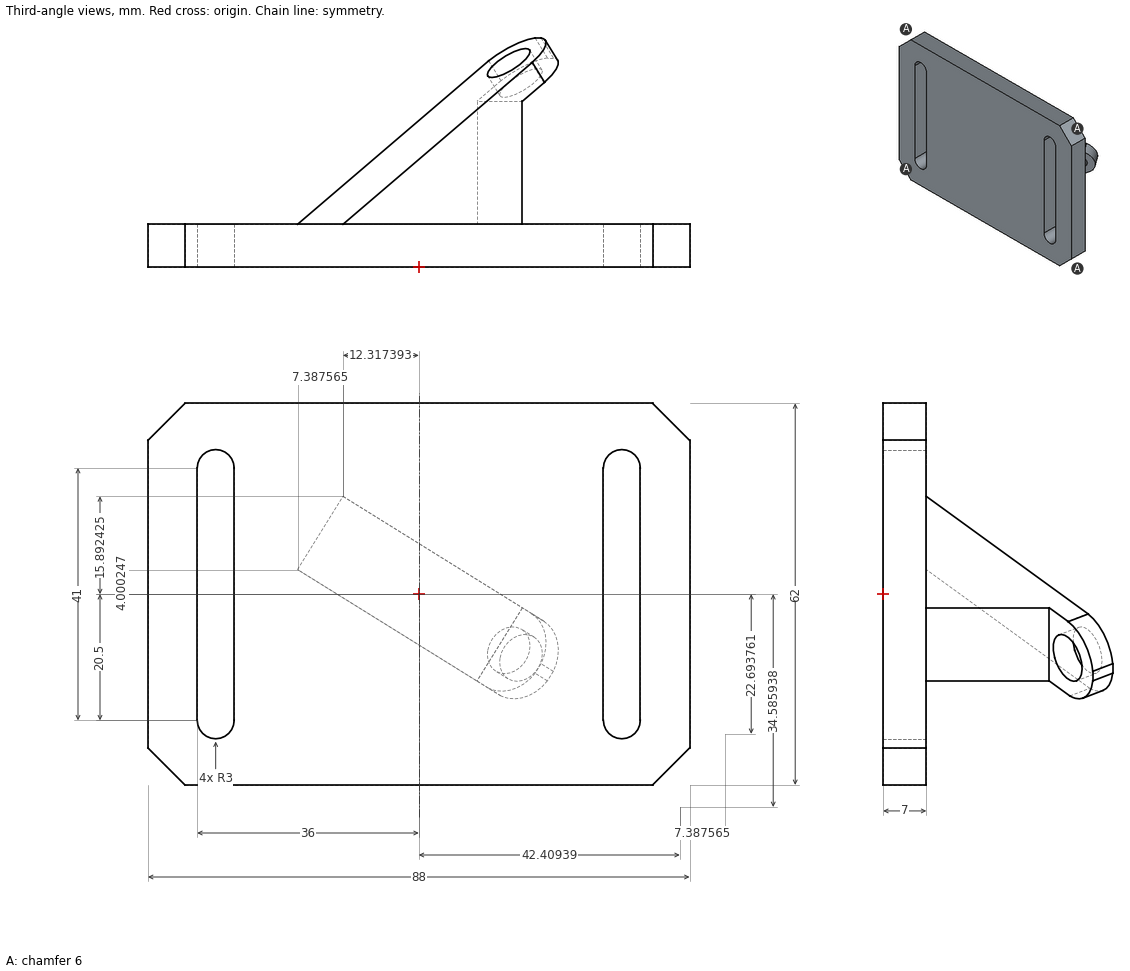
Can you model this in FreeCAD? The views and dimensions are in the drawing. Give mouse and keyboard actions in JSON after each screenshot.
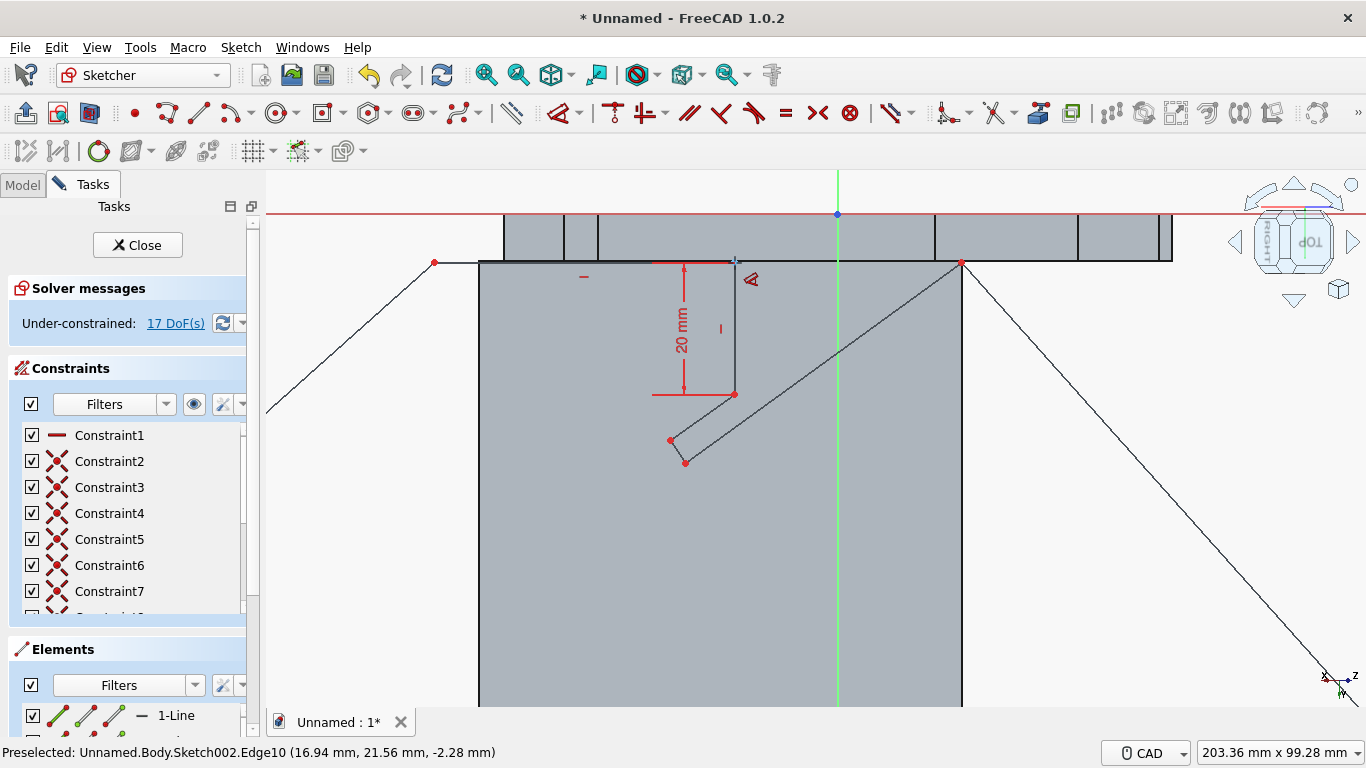
{"action": "left_click", "coordinate": [735, 263]}
{"action": "left_click", "coordinate": [701, 239]}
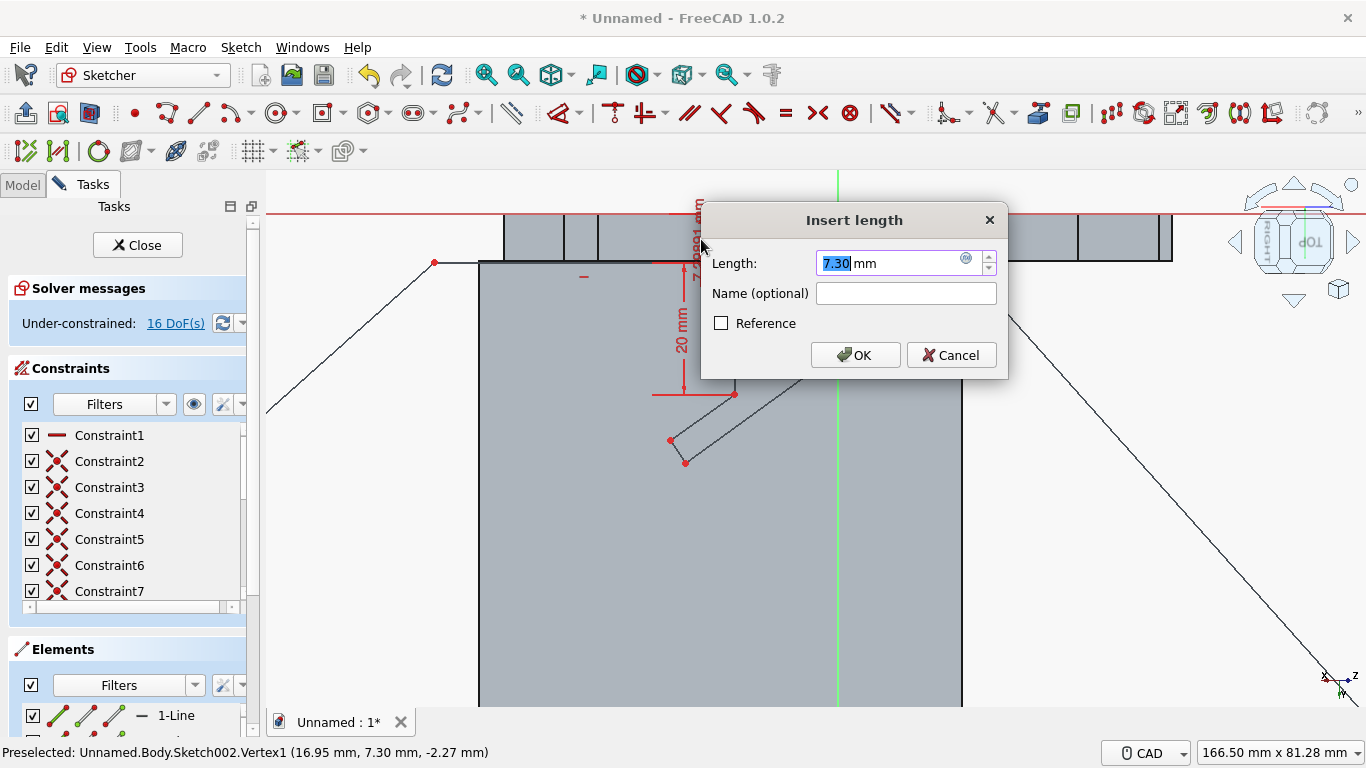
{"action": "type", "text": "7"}
{"action": "key", "text": "Return"}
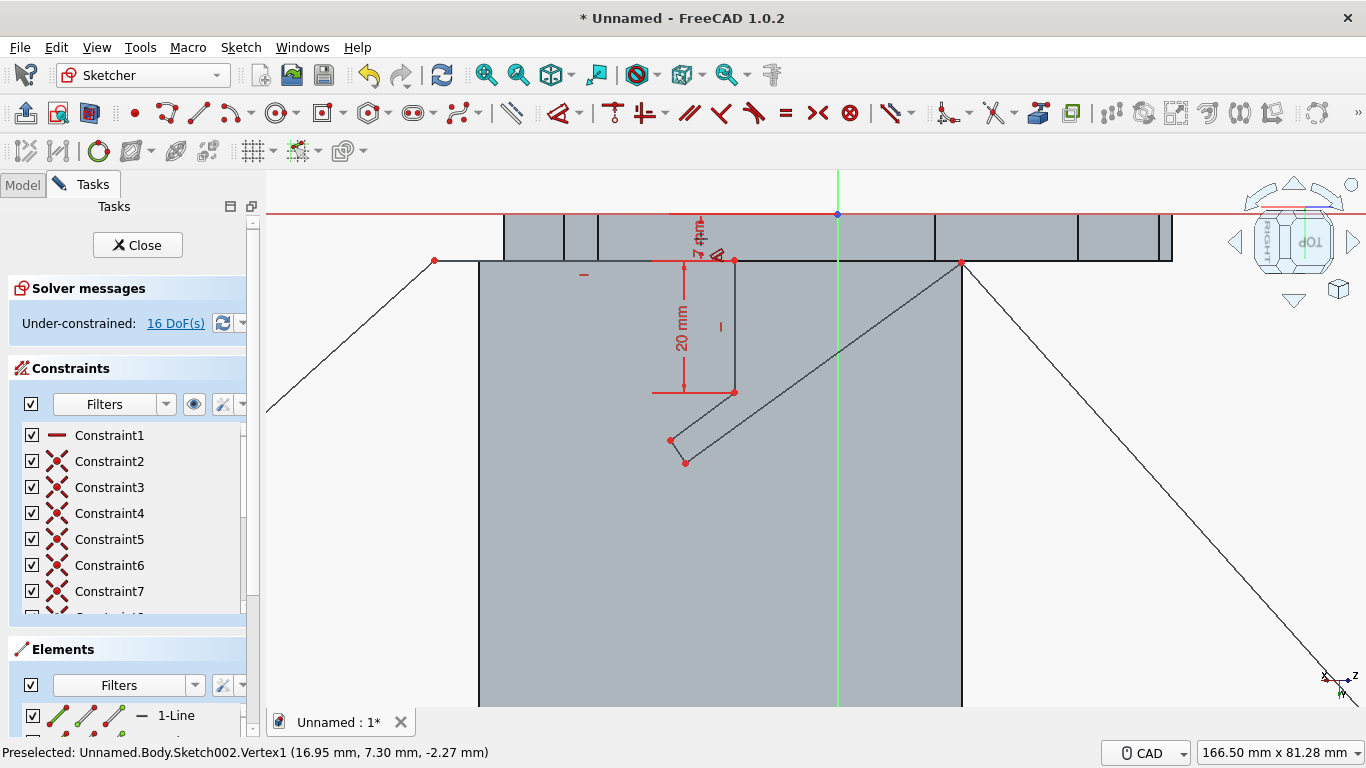
{"action": "left_click", "coordinate": [962, 263]}
{"action": "left_click", "coordinate": [996, 239]}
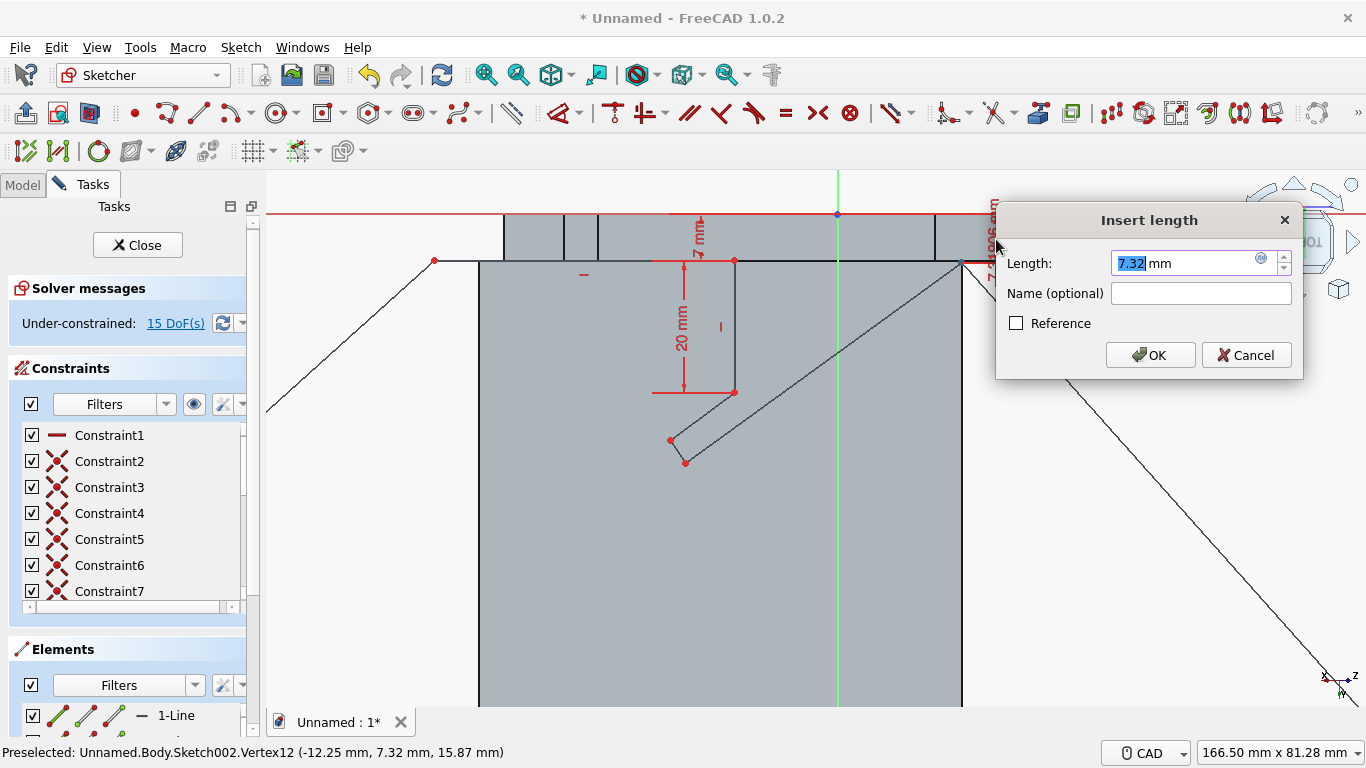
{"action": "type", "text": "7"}
{"action": "key", "text": "Return"}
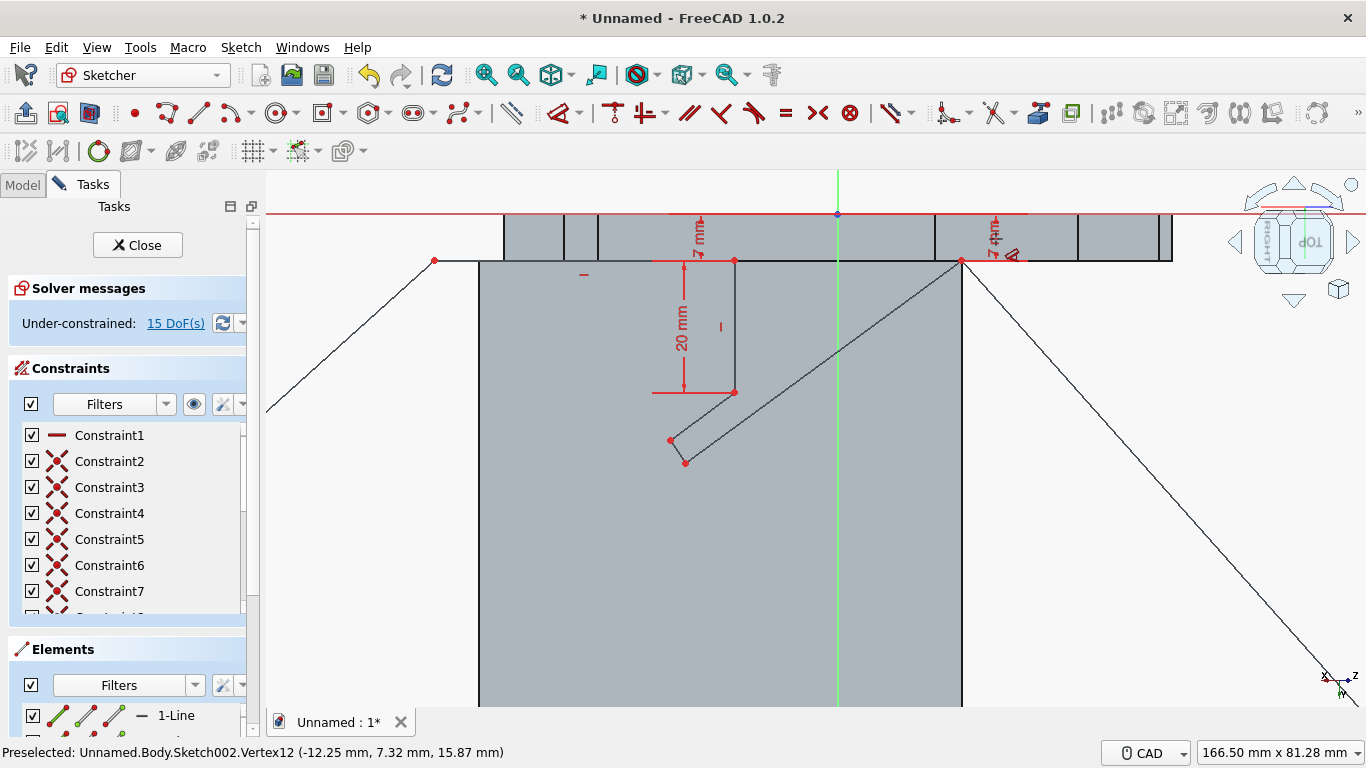
{"action": "left_click", "coordinate": [645, 261]}
{"action": "left_click", "coordinate": [585, 295]}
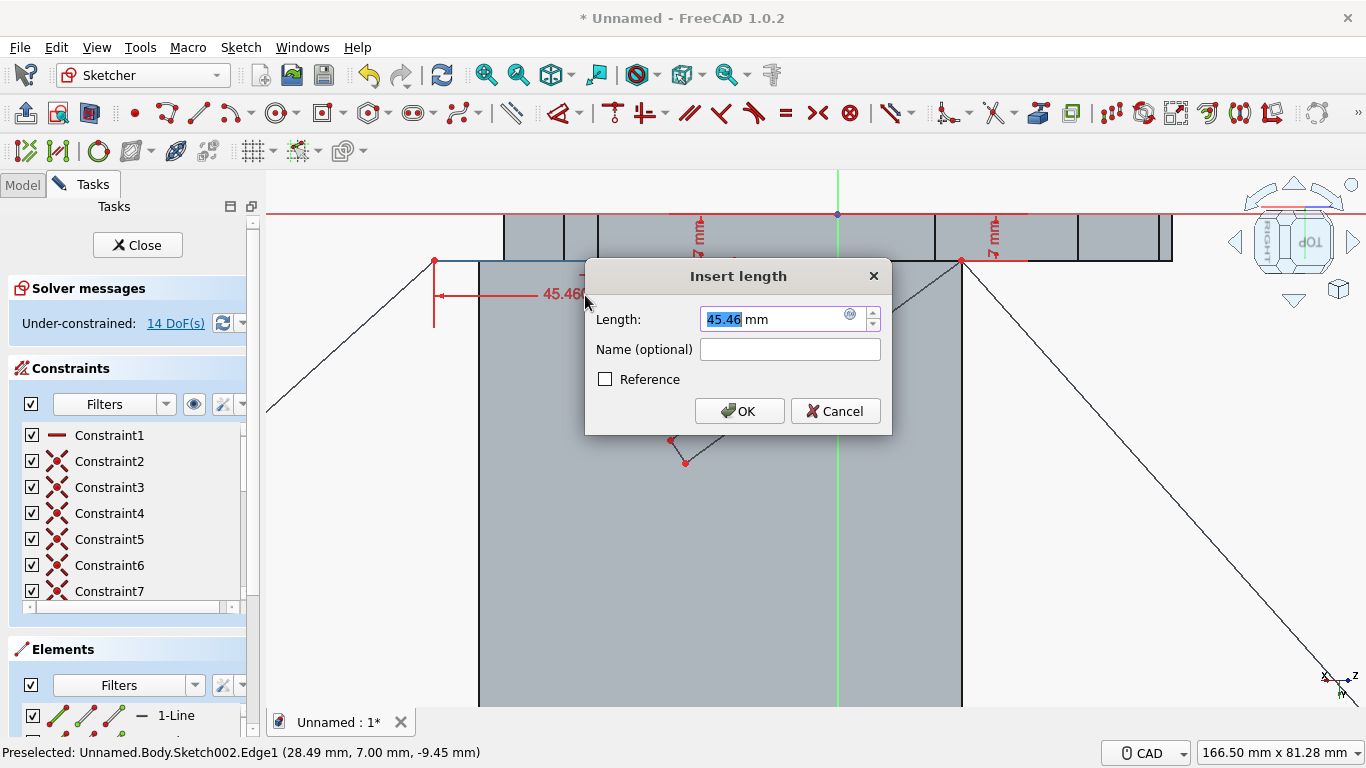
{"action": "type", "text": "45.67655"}
{"action": "key", "text": "Return"}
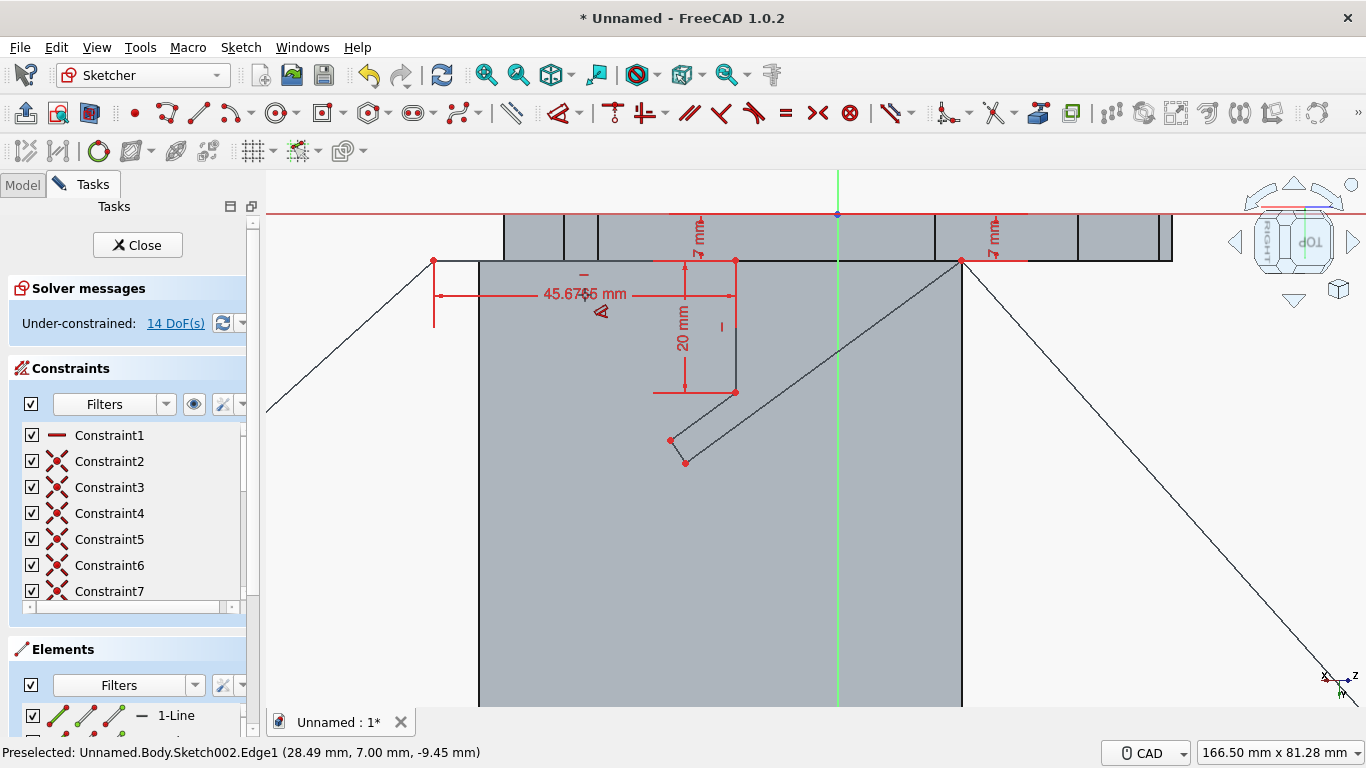
{"action": "scroll", "coordinate": [709, 334], "scroll_direction": "down", "scroll_amount": 4}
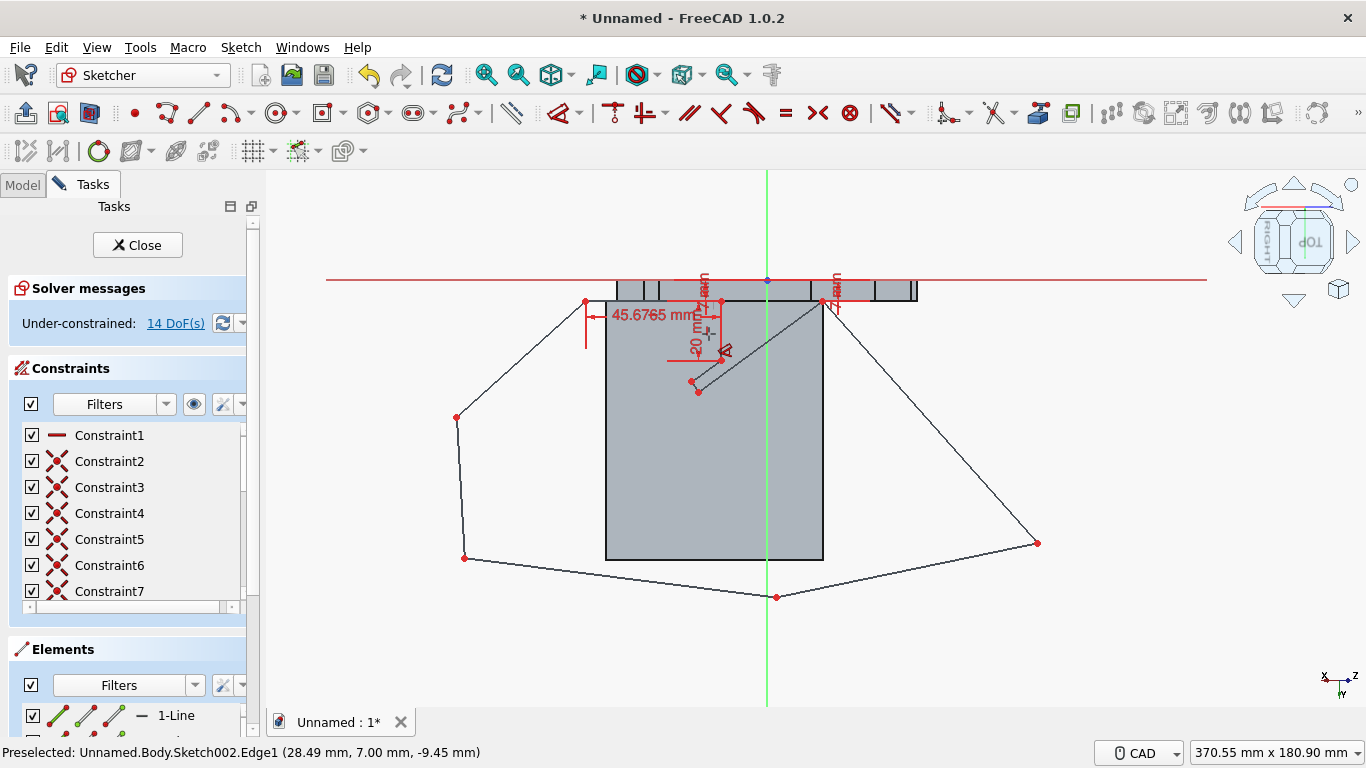
{"action": "scroll", "coordinate": [459, 459], "scroll_direction": "up", "scroll_amount": 11}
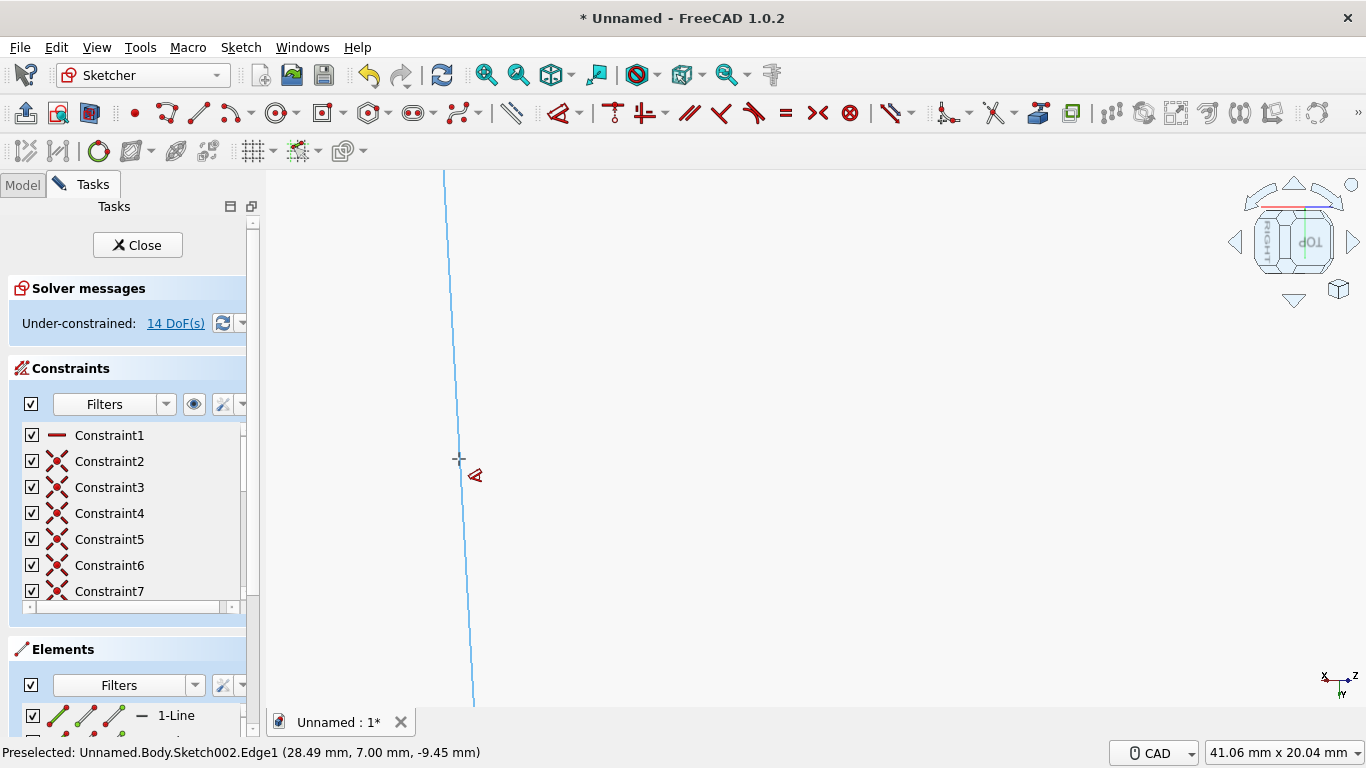
{"action": "left_click", "coordinate": [460, 459]}